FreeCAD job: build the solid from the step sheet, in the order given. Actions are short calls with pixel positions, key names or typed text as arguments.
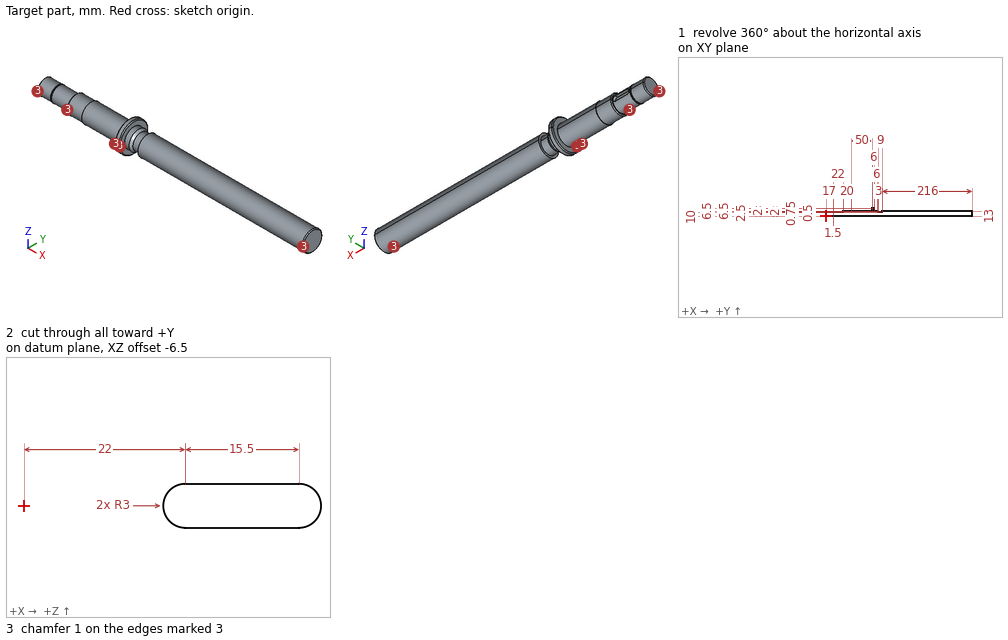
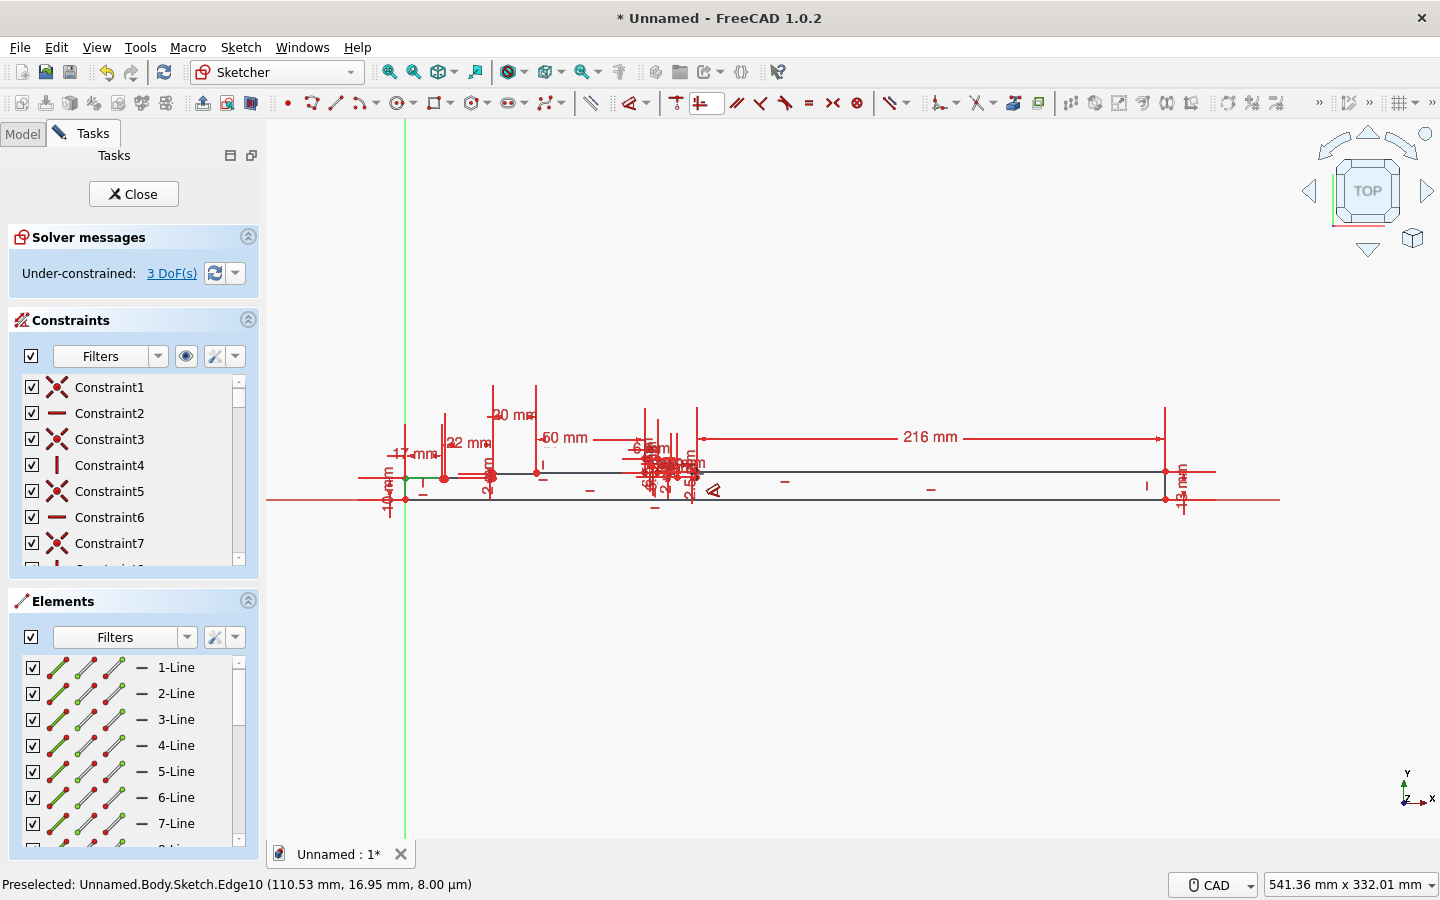
scroll(536, 473, up, 19)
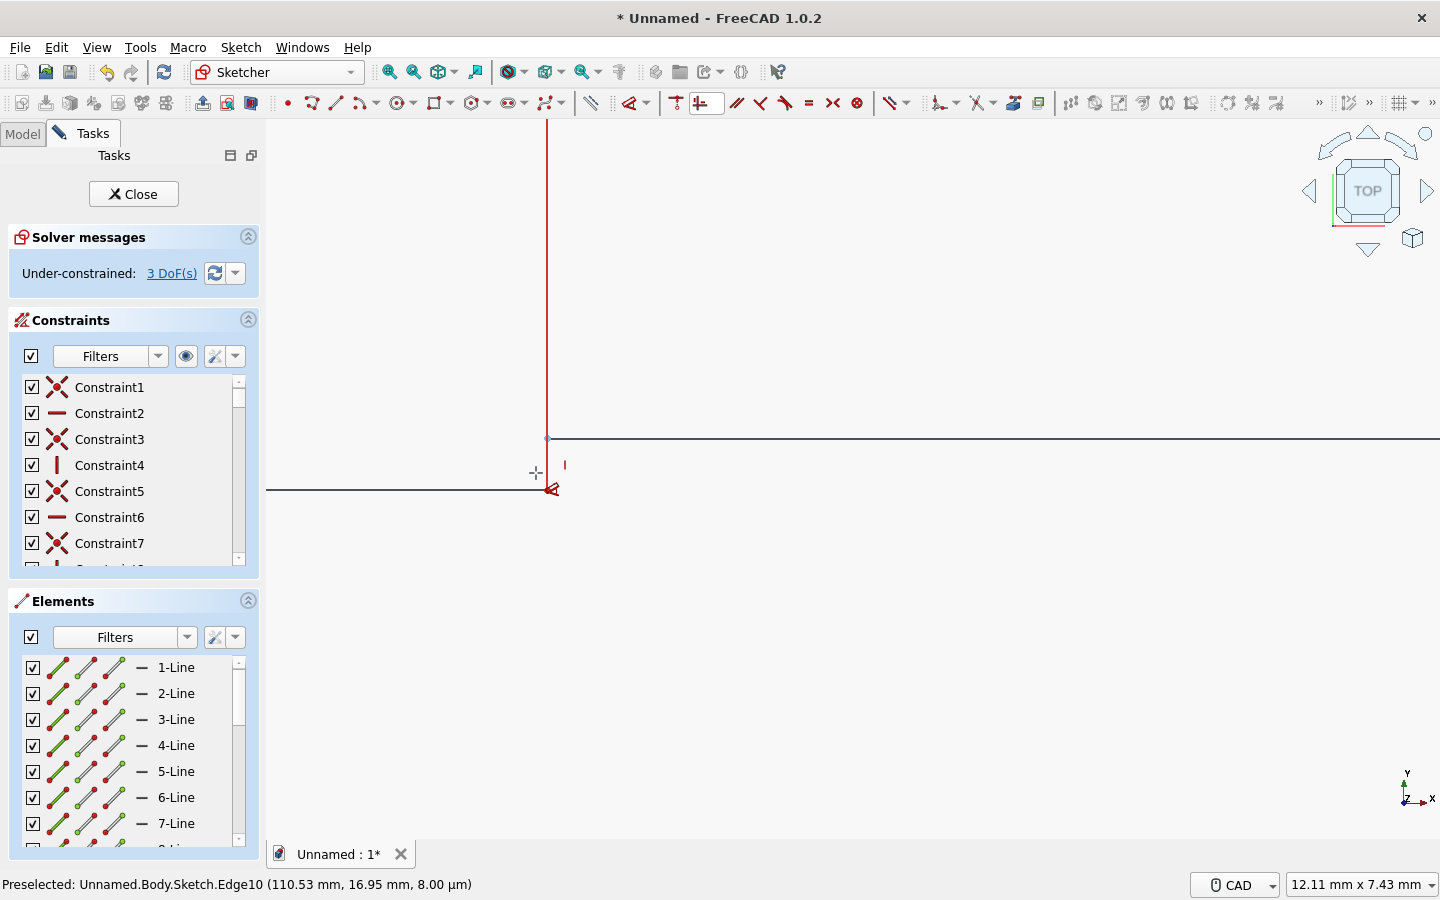
click(547, 465)
click(513, 465)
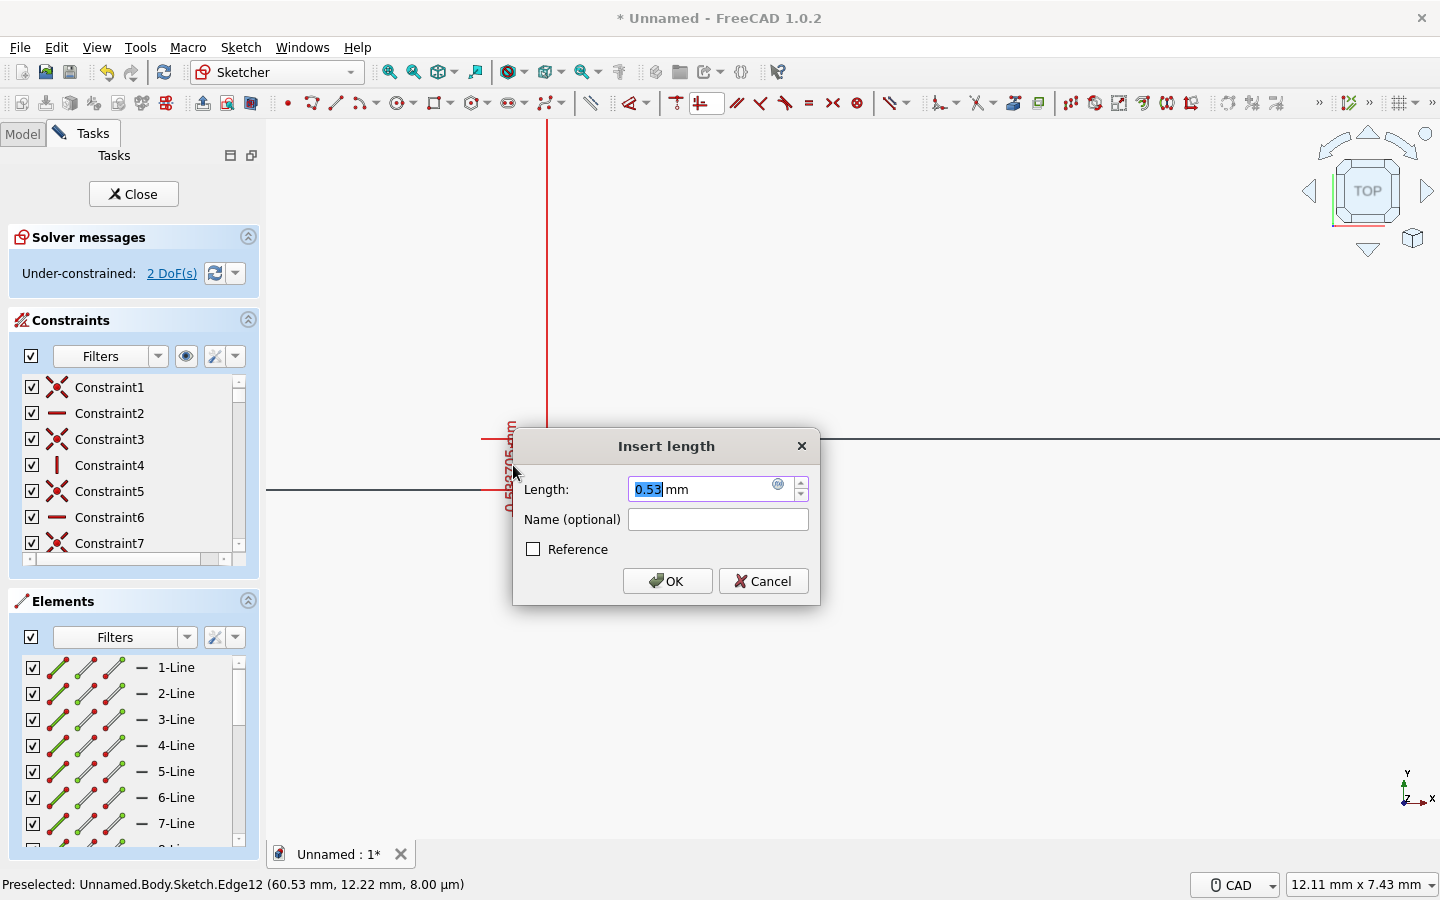
text(0.5)
key(Return)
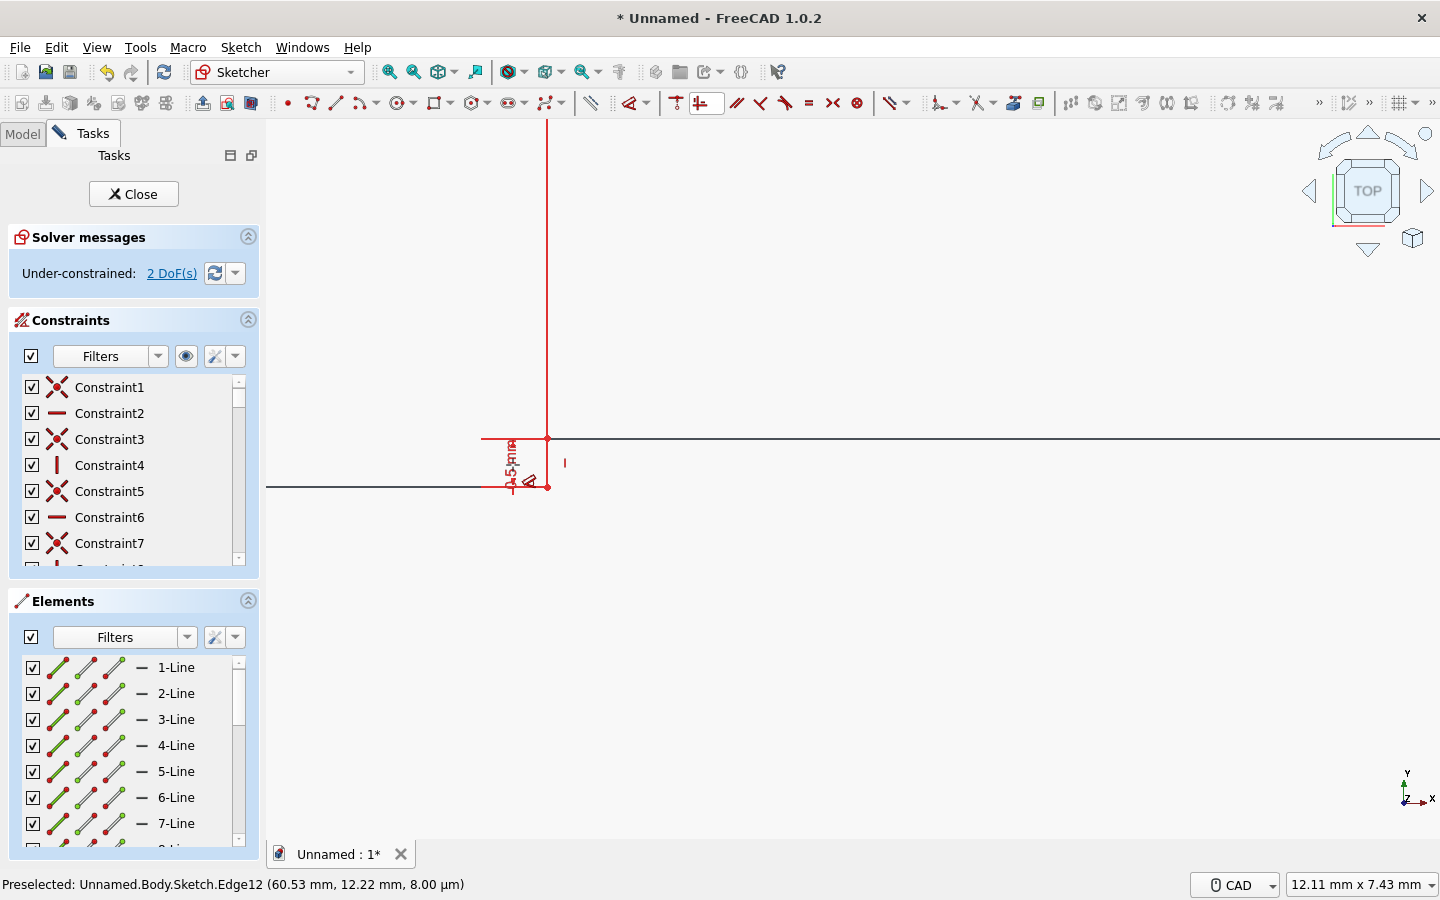
scroll(479, 472, down, 18)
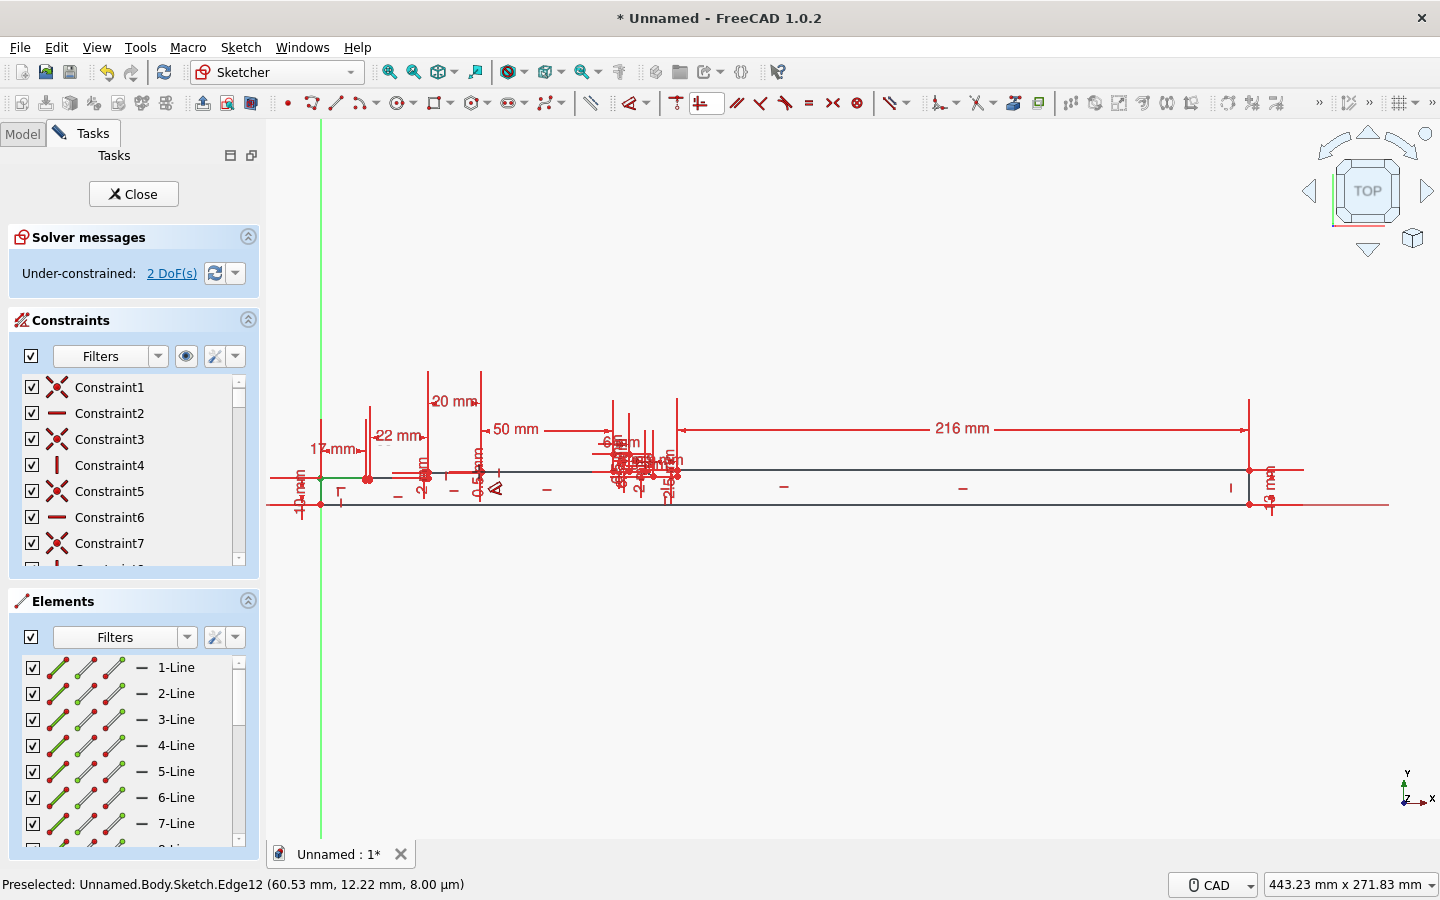
scroll(369, 480, up, 13)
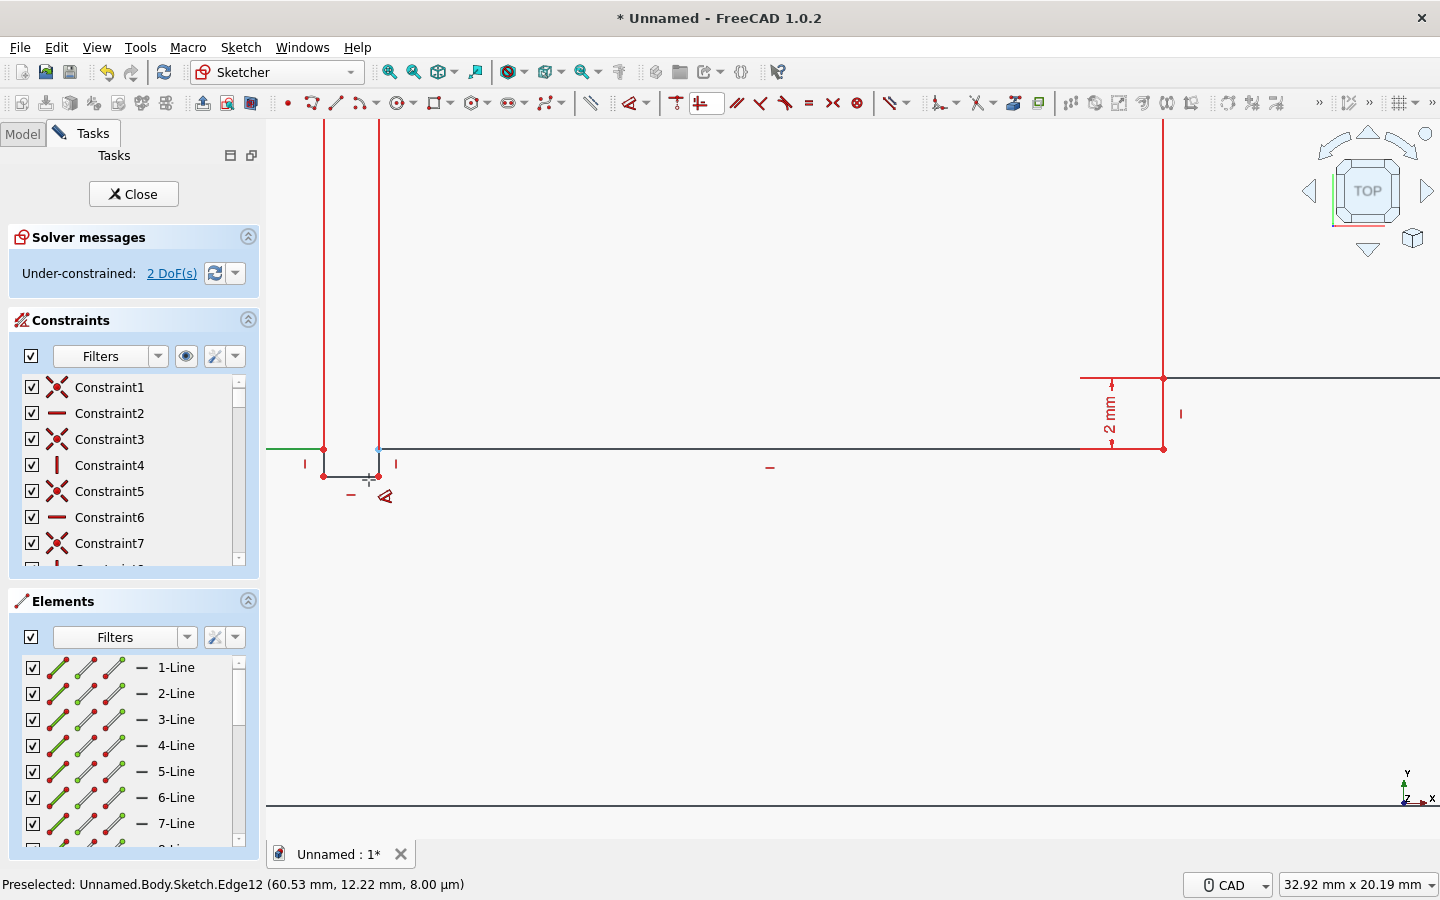
click(362, 477)
click(351, 511)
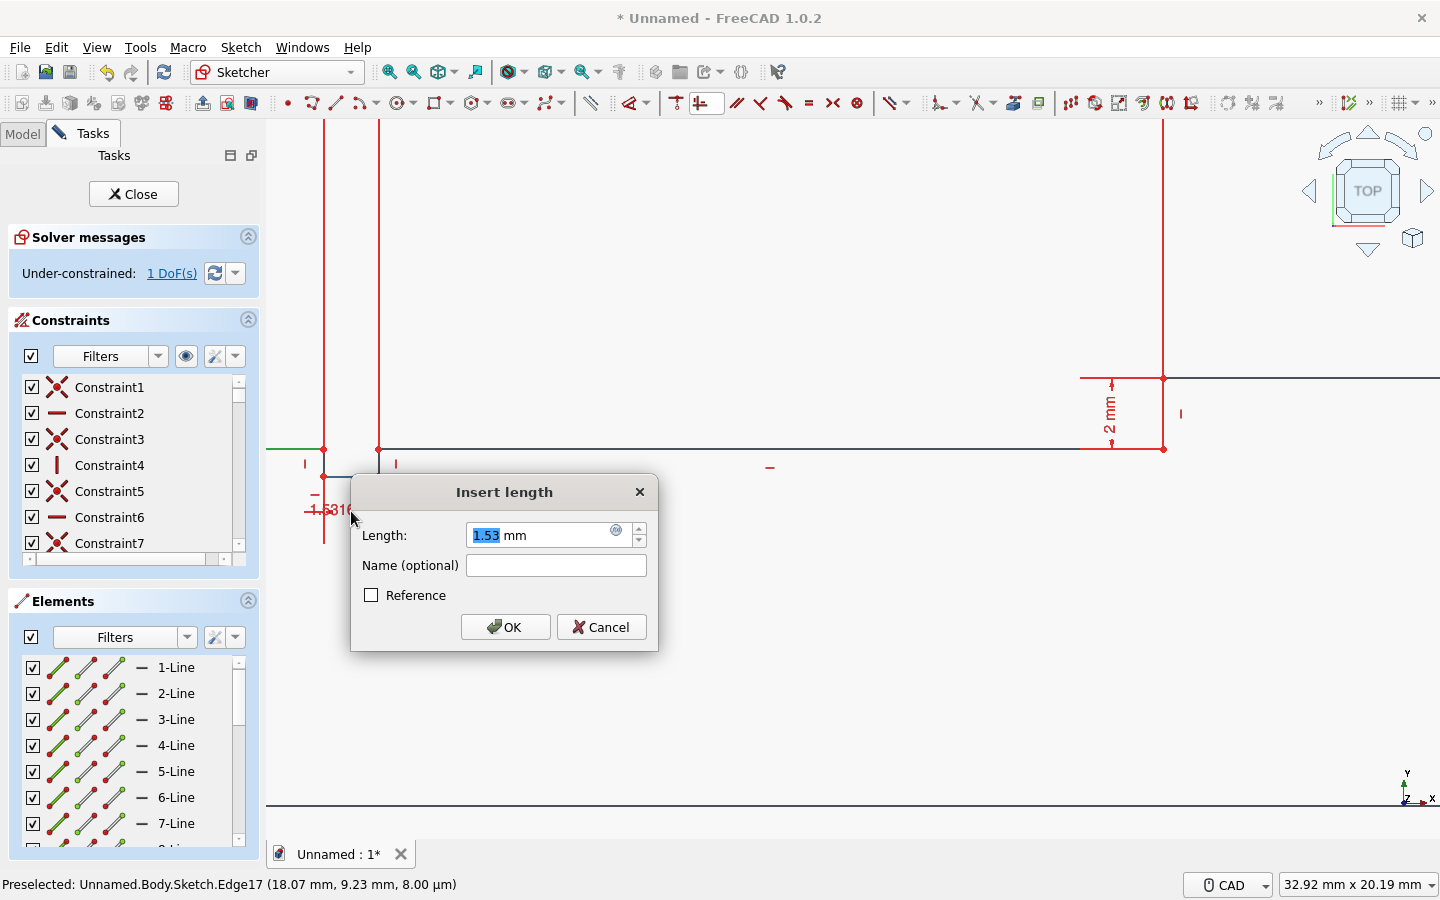
text(1.5)
key(Return)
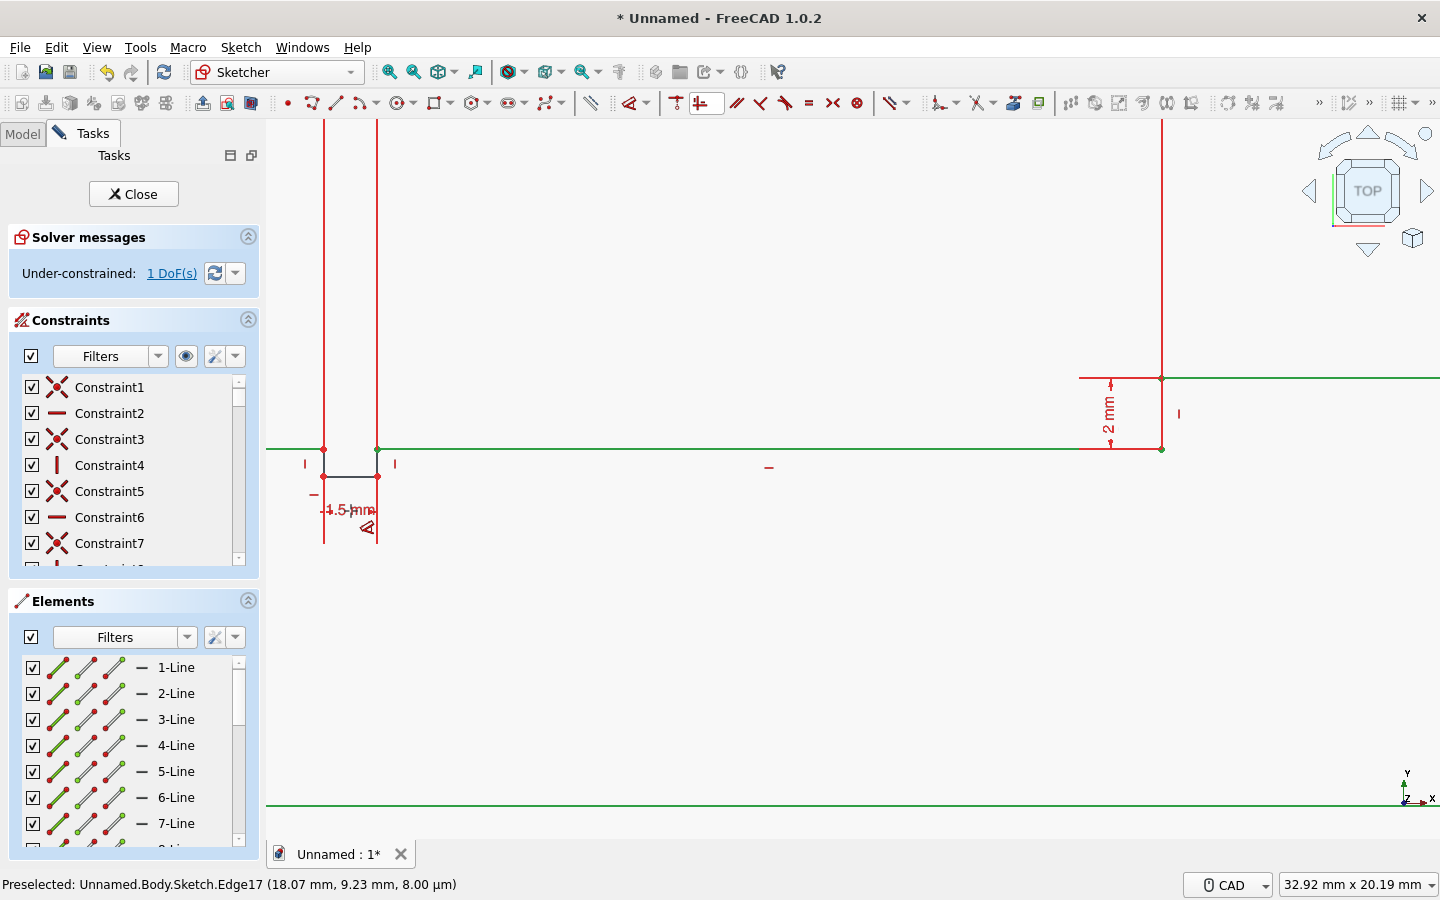
scroll(377, 460, up, 2)